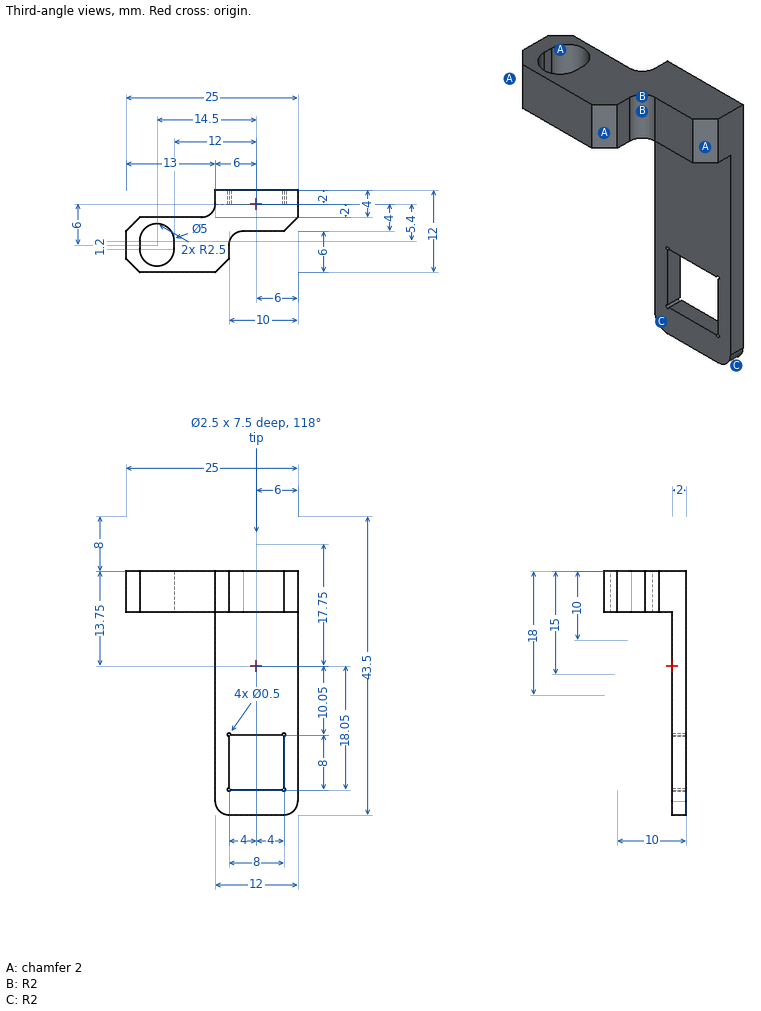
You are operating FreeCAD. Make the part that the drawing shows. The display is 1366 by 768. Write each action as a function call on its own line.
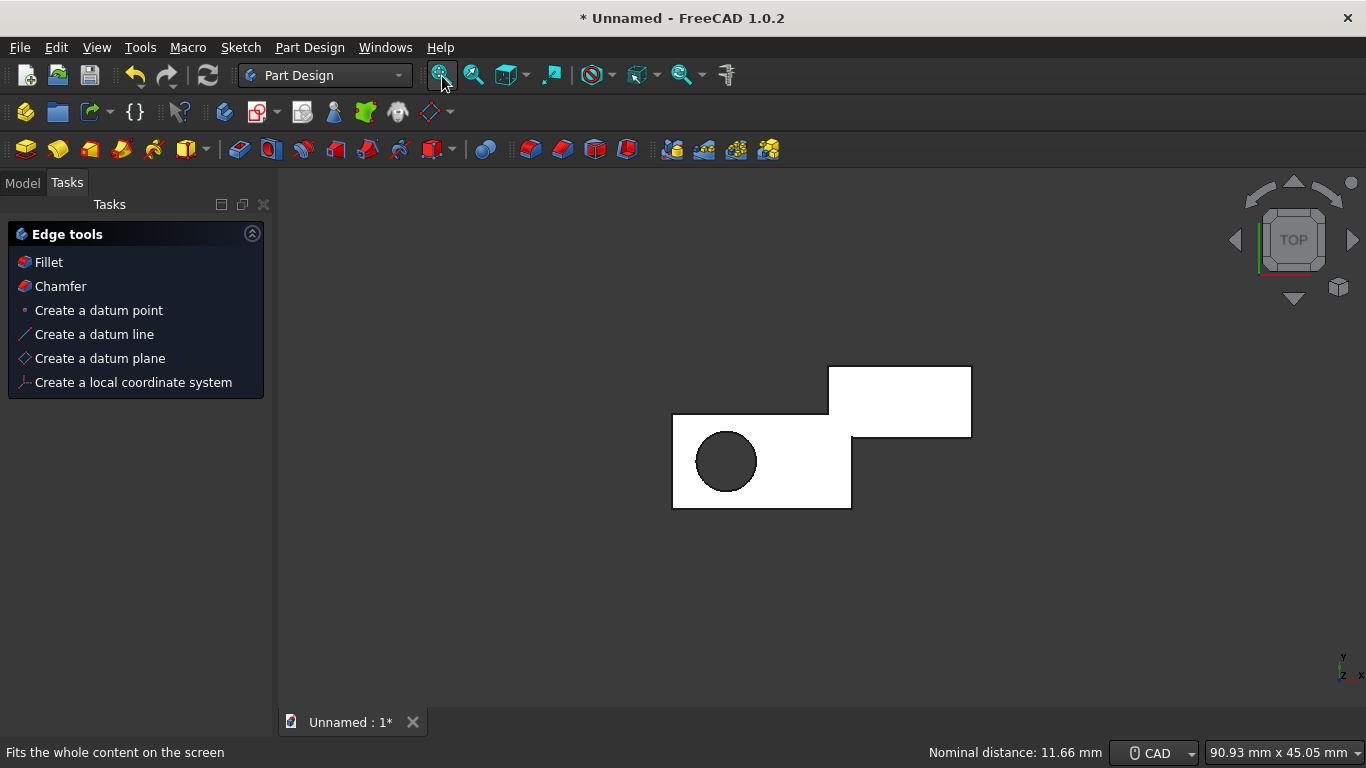
key(0)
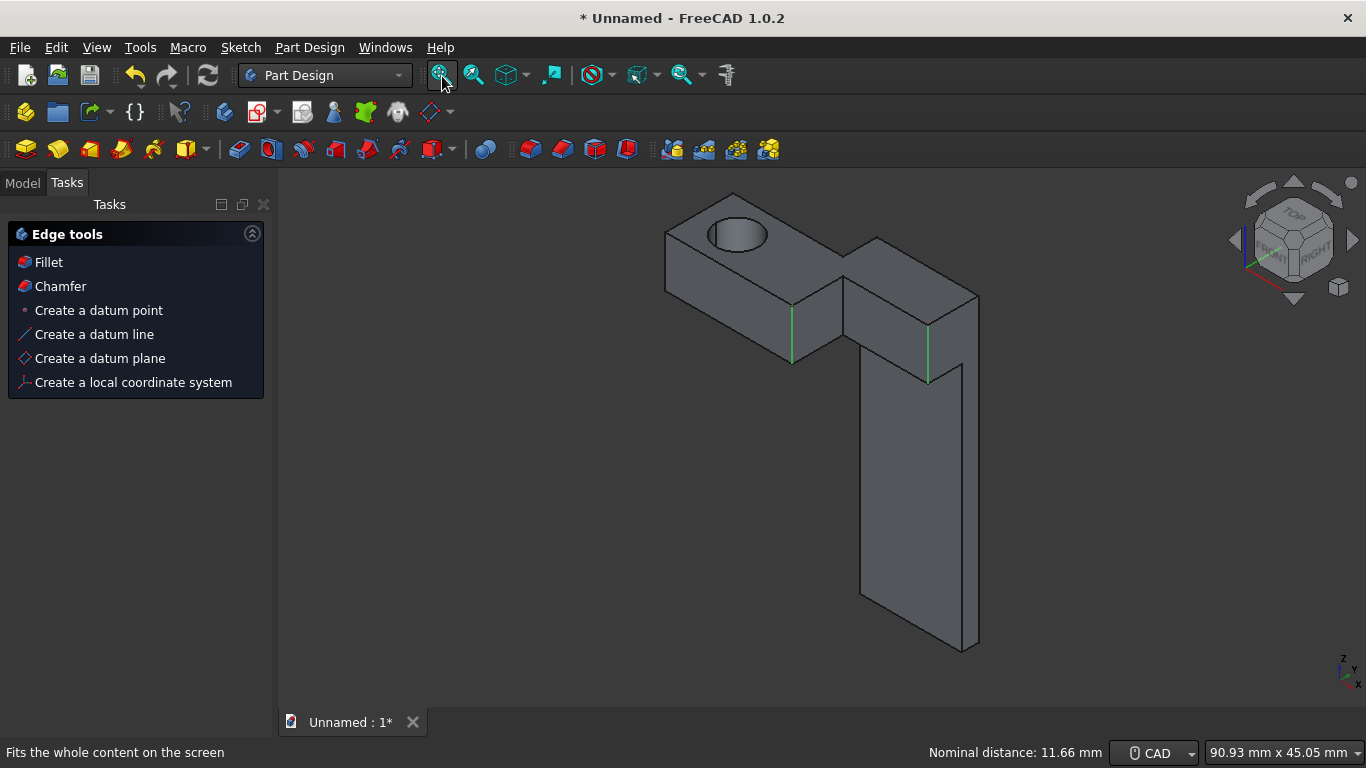
key(1)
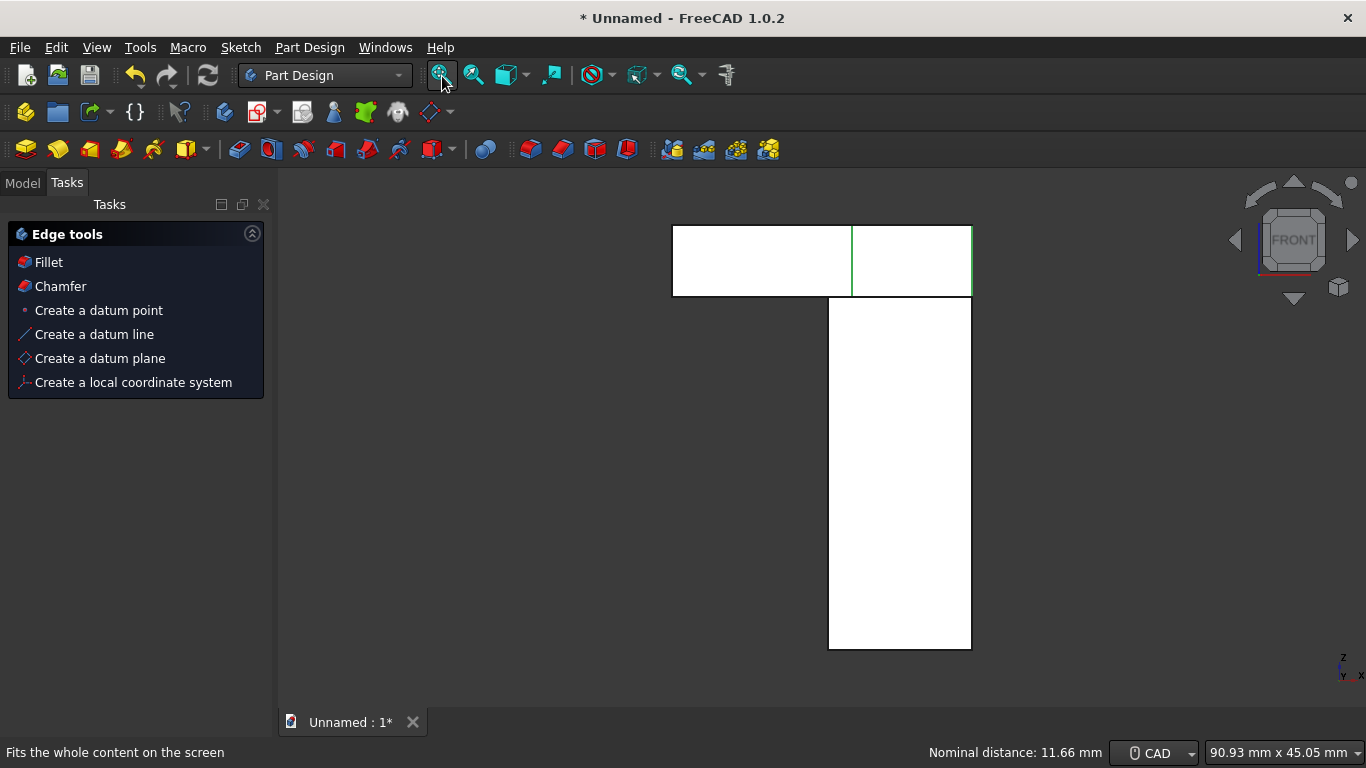
click(672, 260, ctrl)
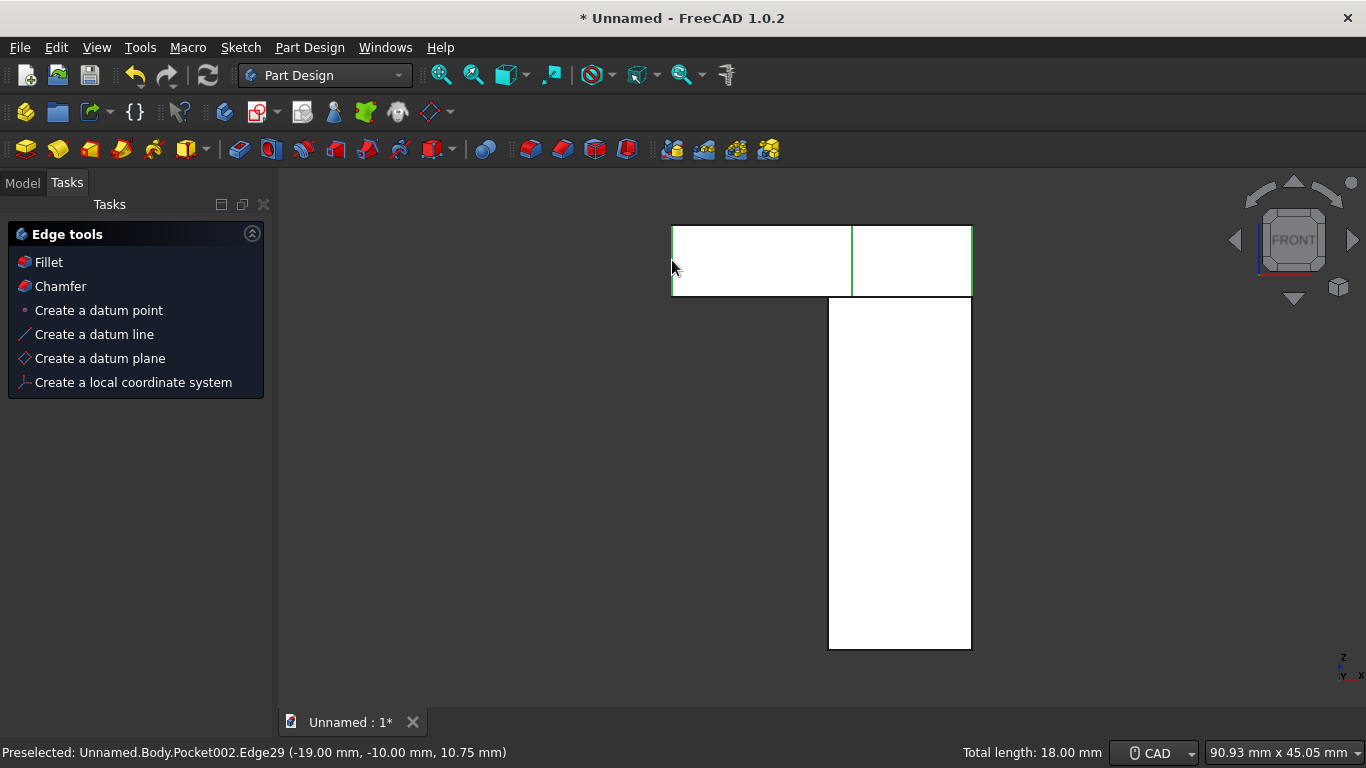
key(3)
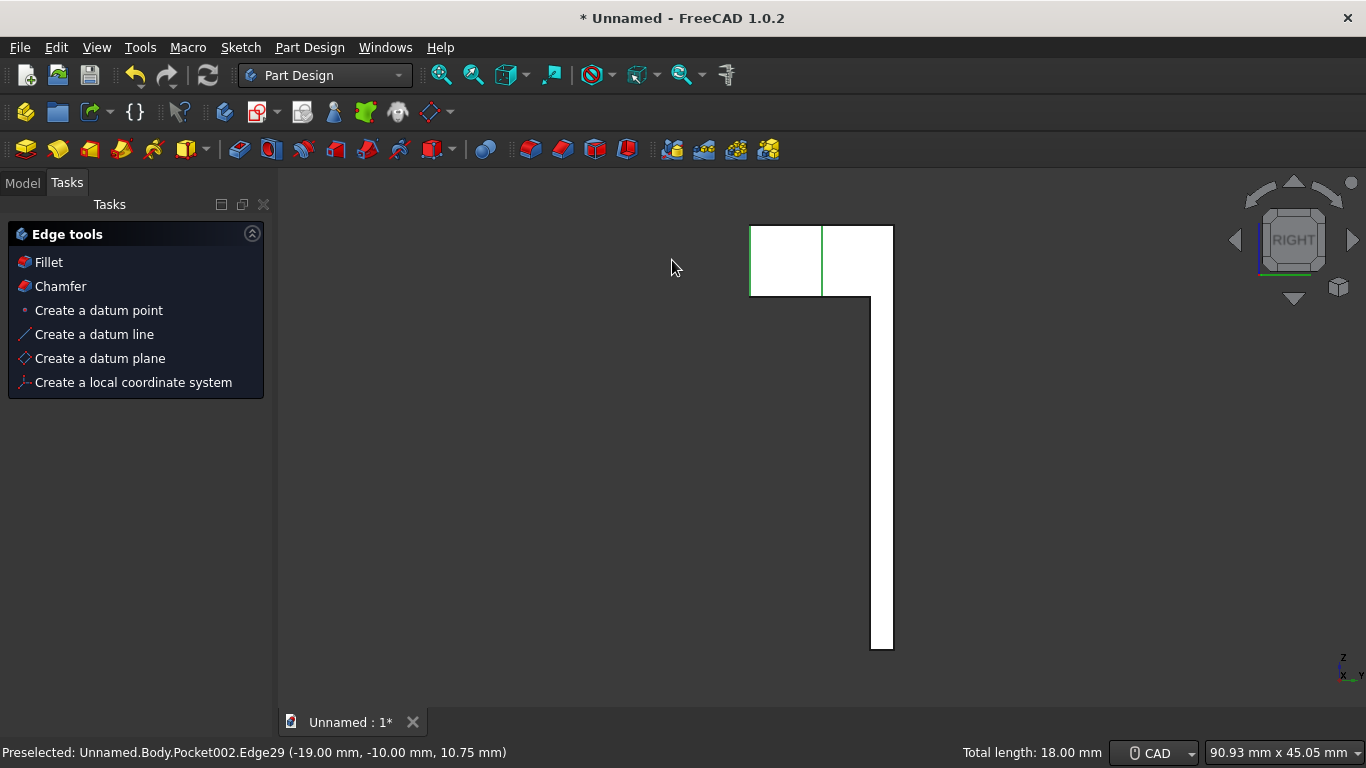
key(5)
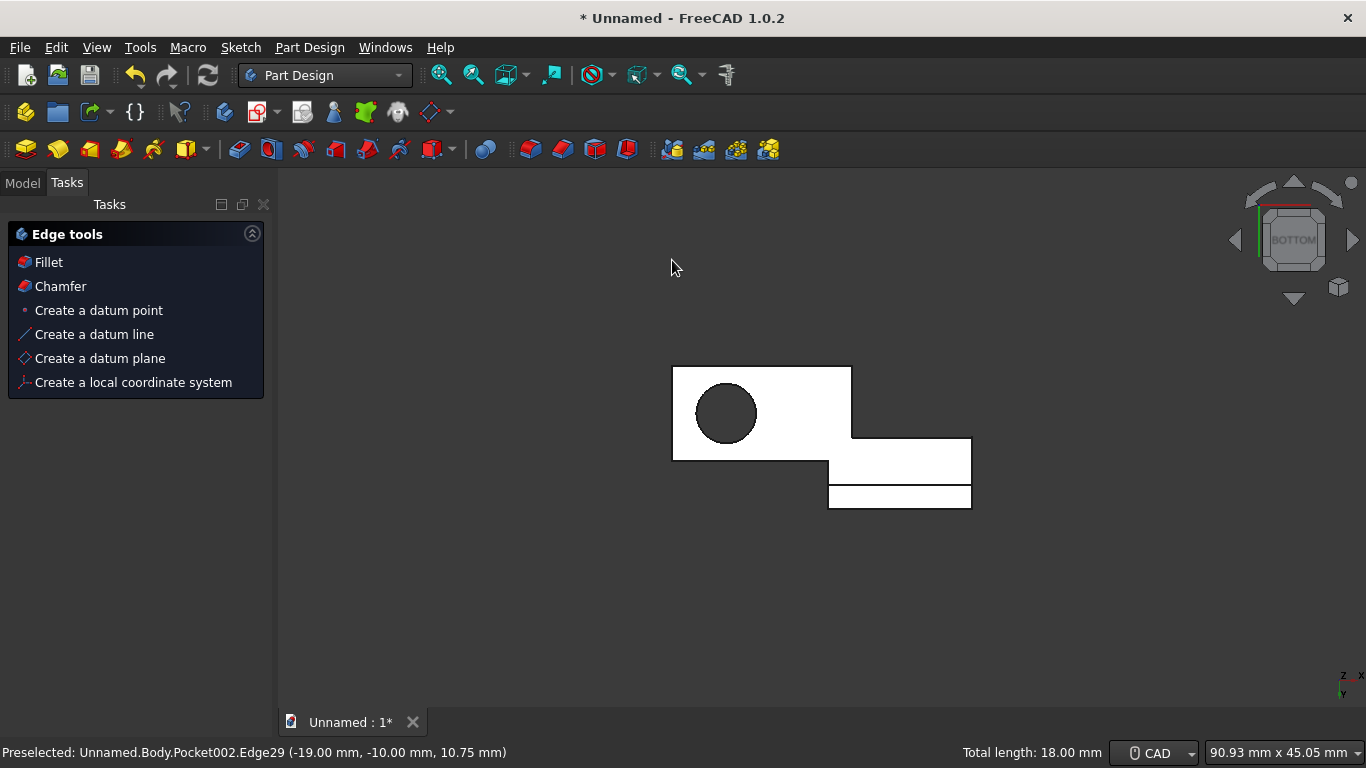
click(442, 76)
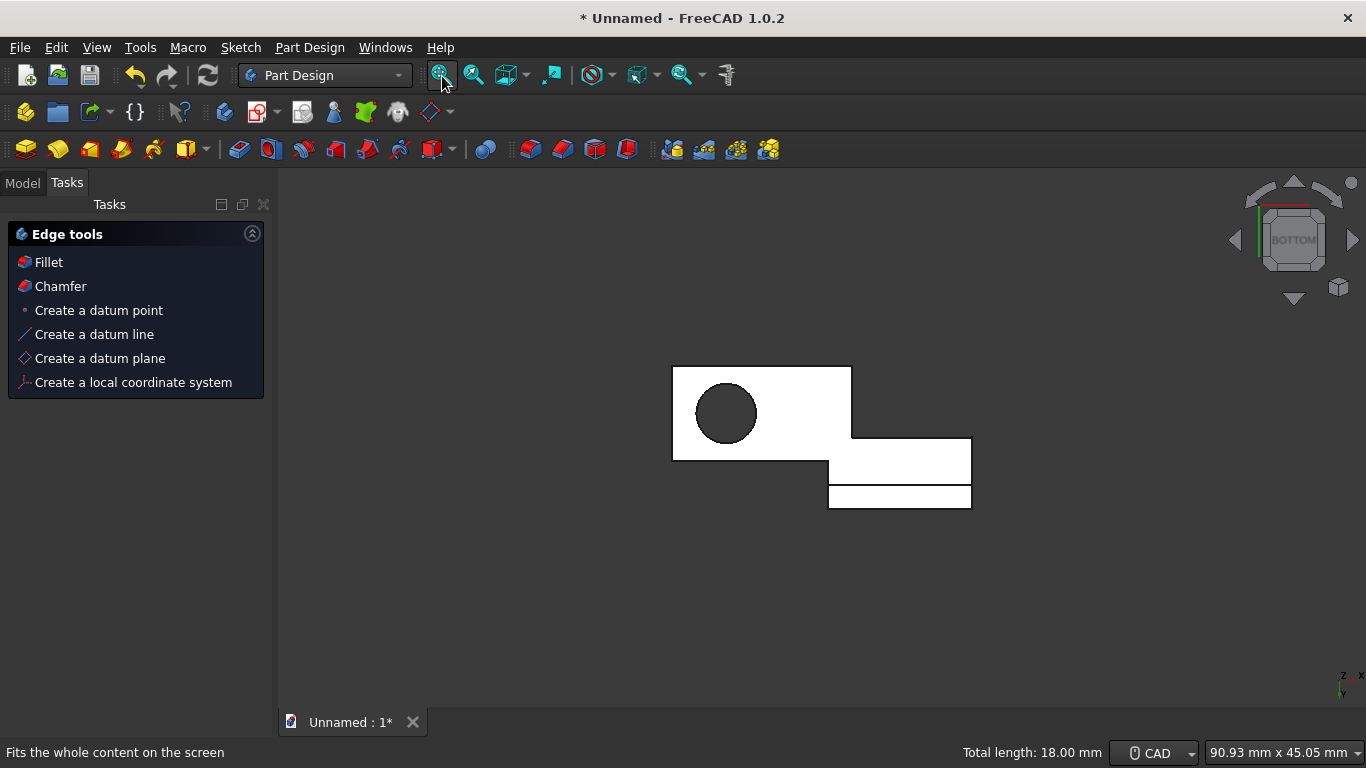
key(4)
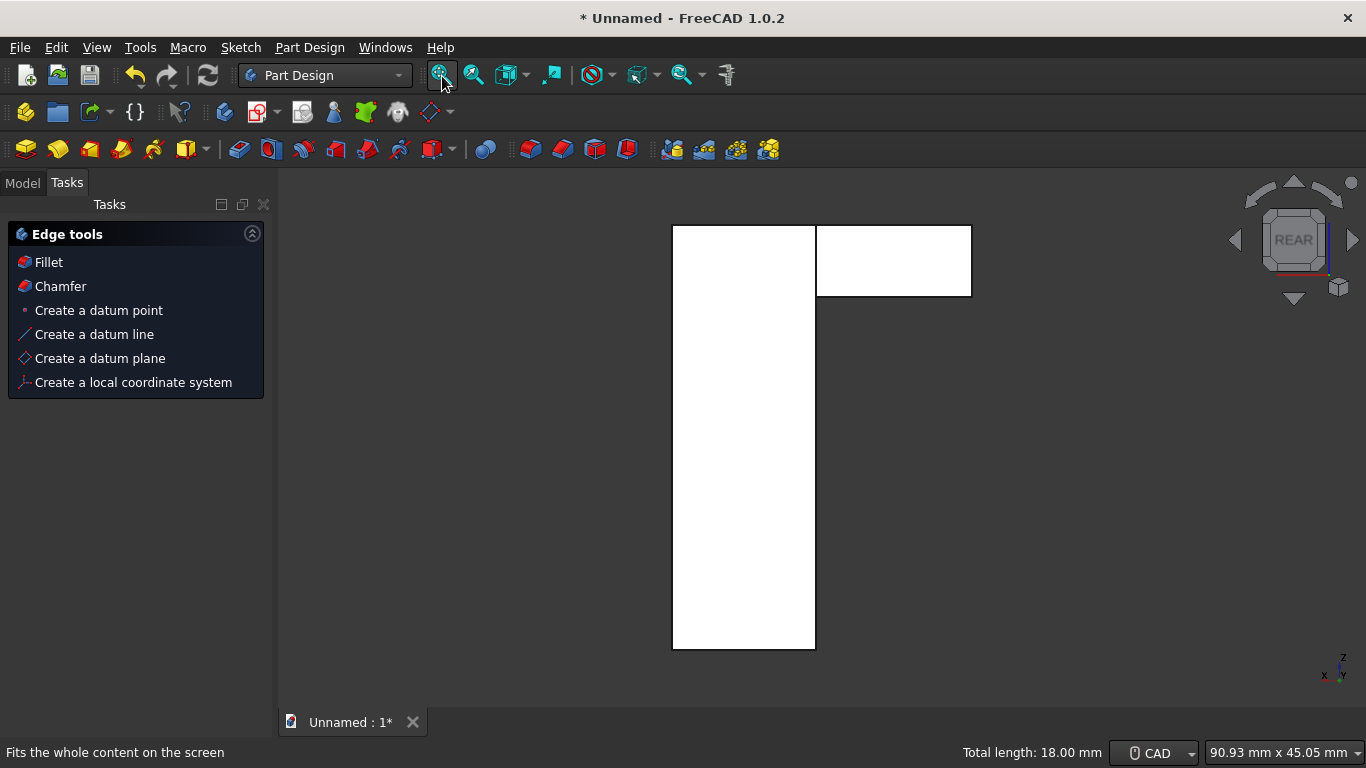
click(972, 260, ctrl)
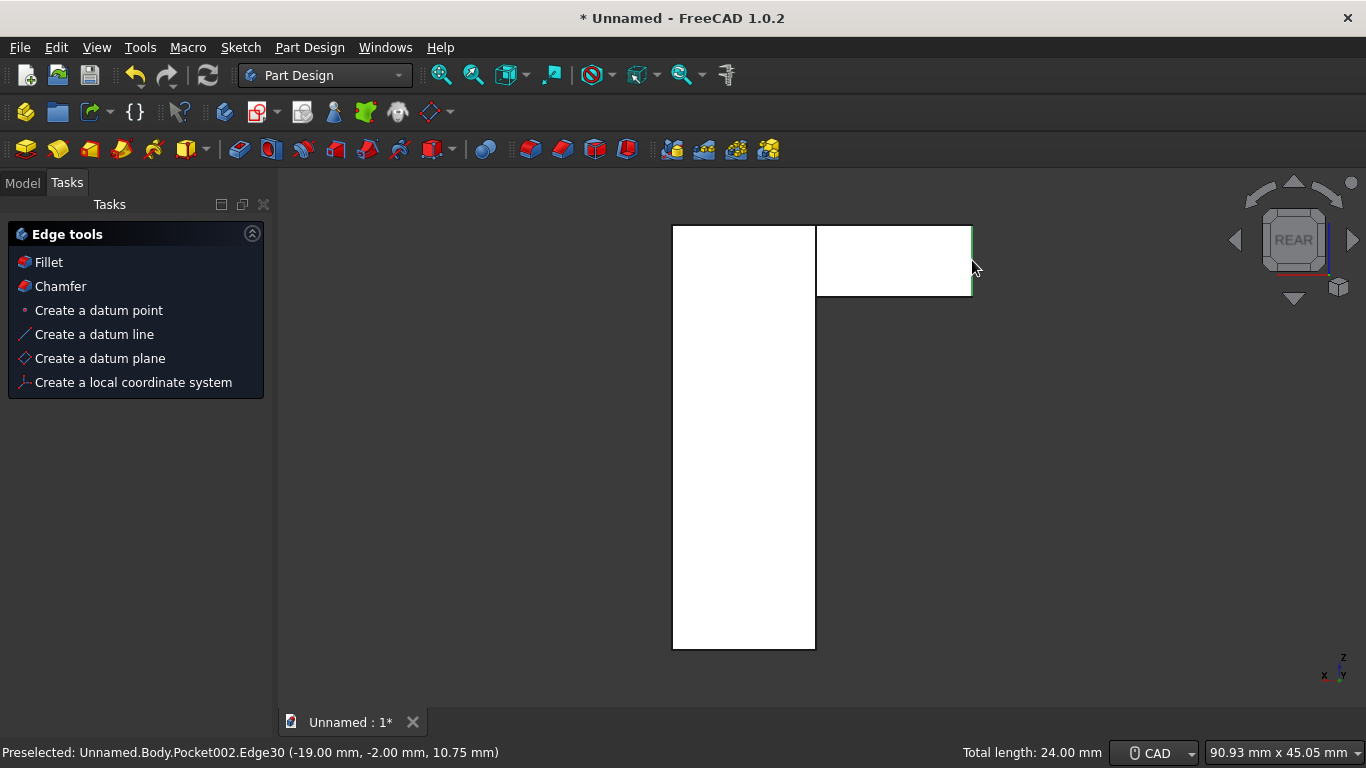
click(564, 150)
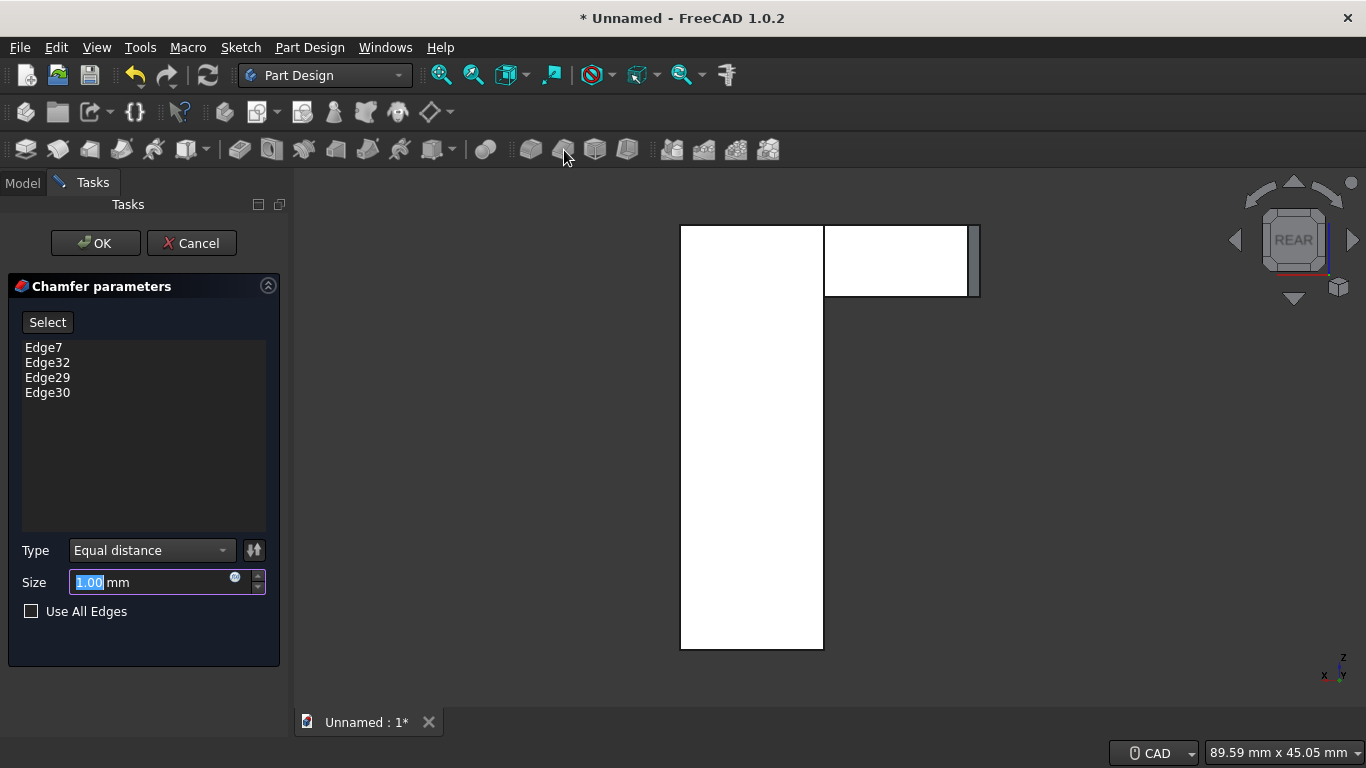
text(2)
key(Tab)